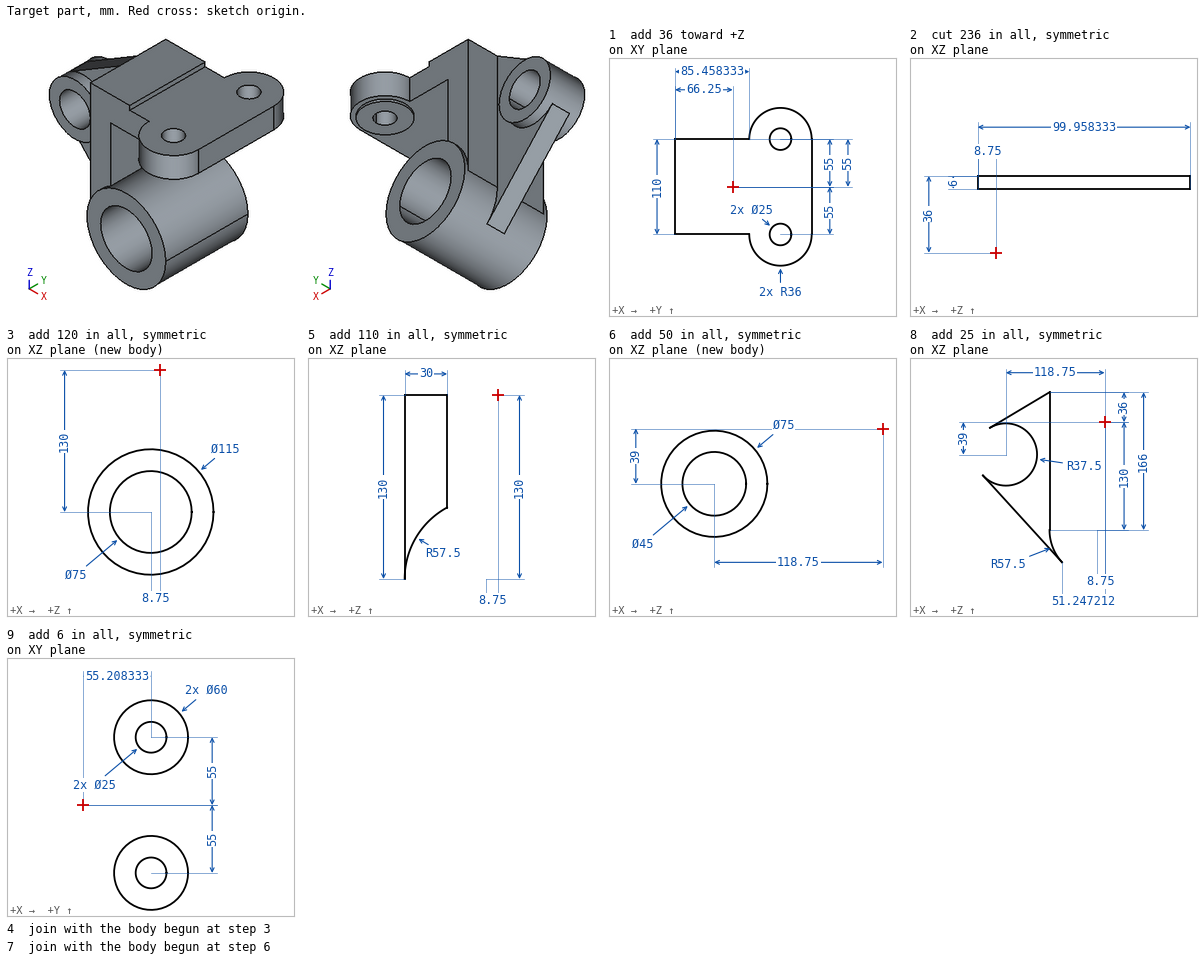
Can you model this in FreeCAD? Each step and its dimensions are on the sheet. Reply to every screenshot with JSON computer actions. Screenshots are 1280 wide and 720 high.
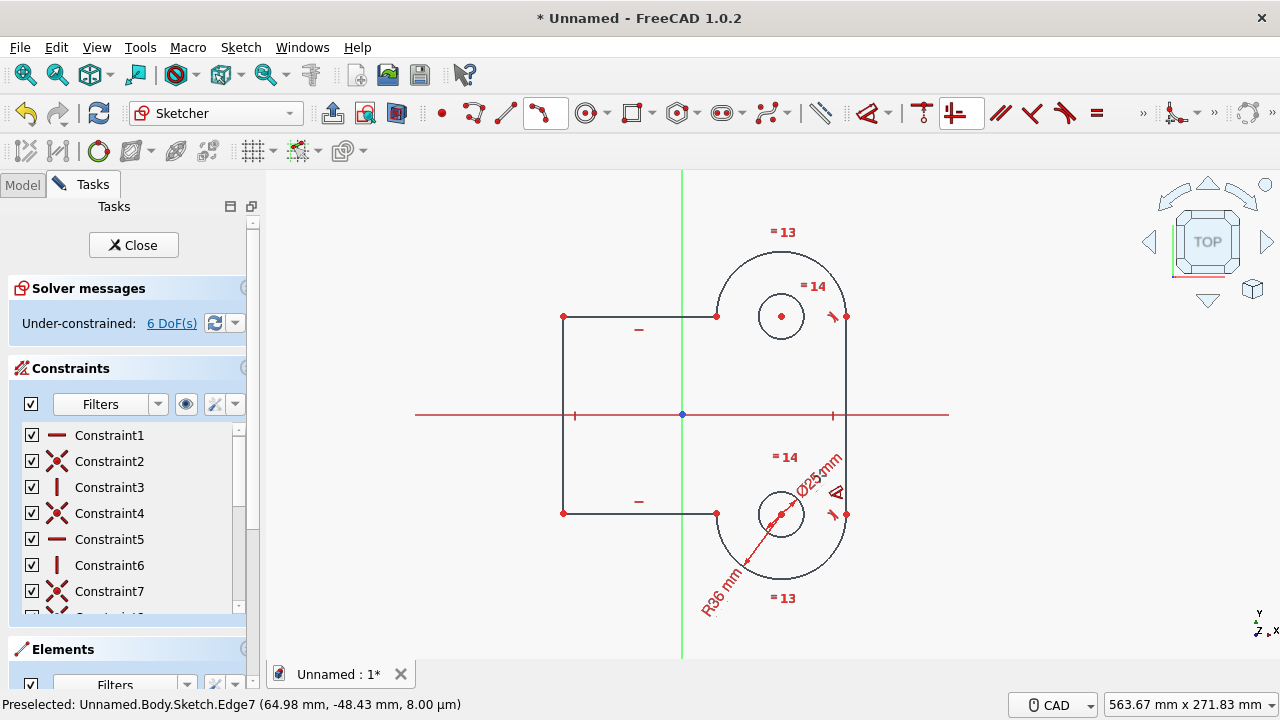
{"action": "left_click", "coordinate": [781, 514]}
{"action": "left_click", "coordinate": [815, 441]}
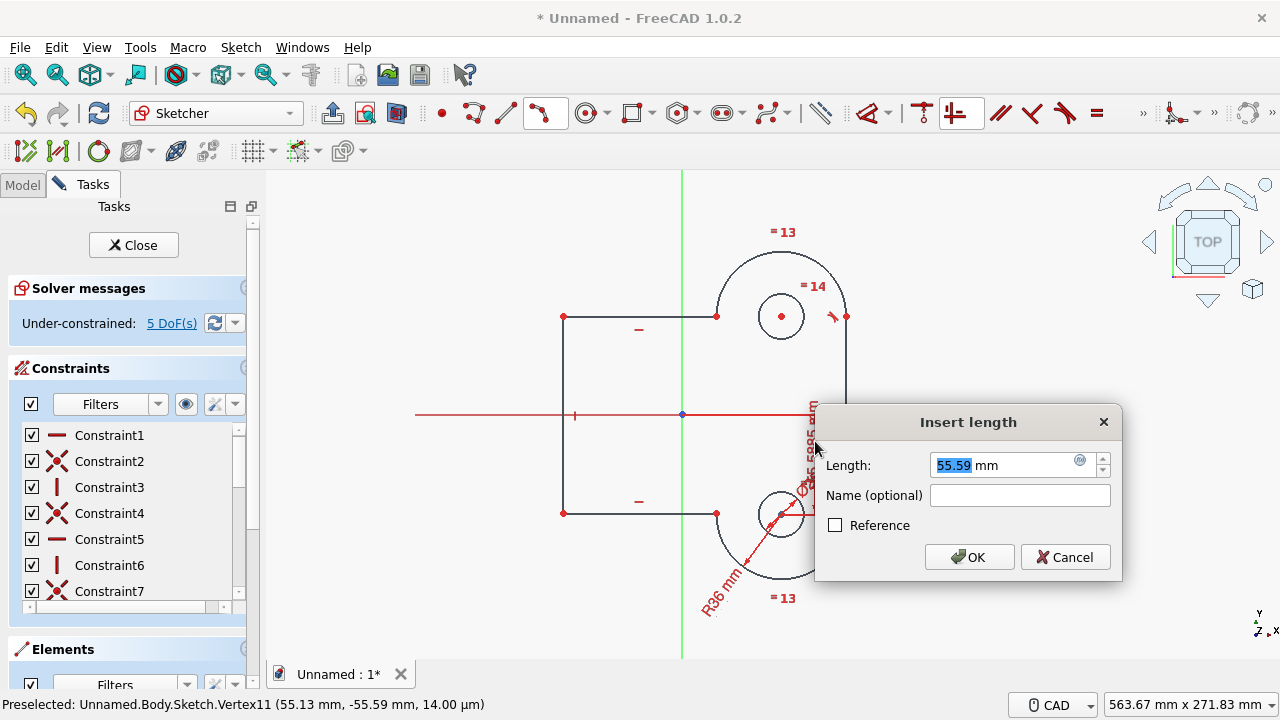
{"action": "type", "text": "55"}
{"action": "key", "text": "Return"}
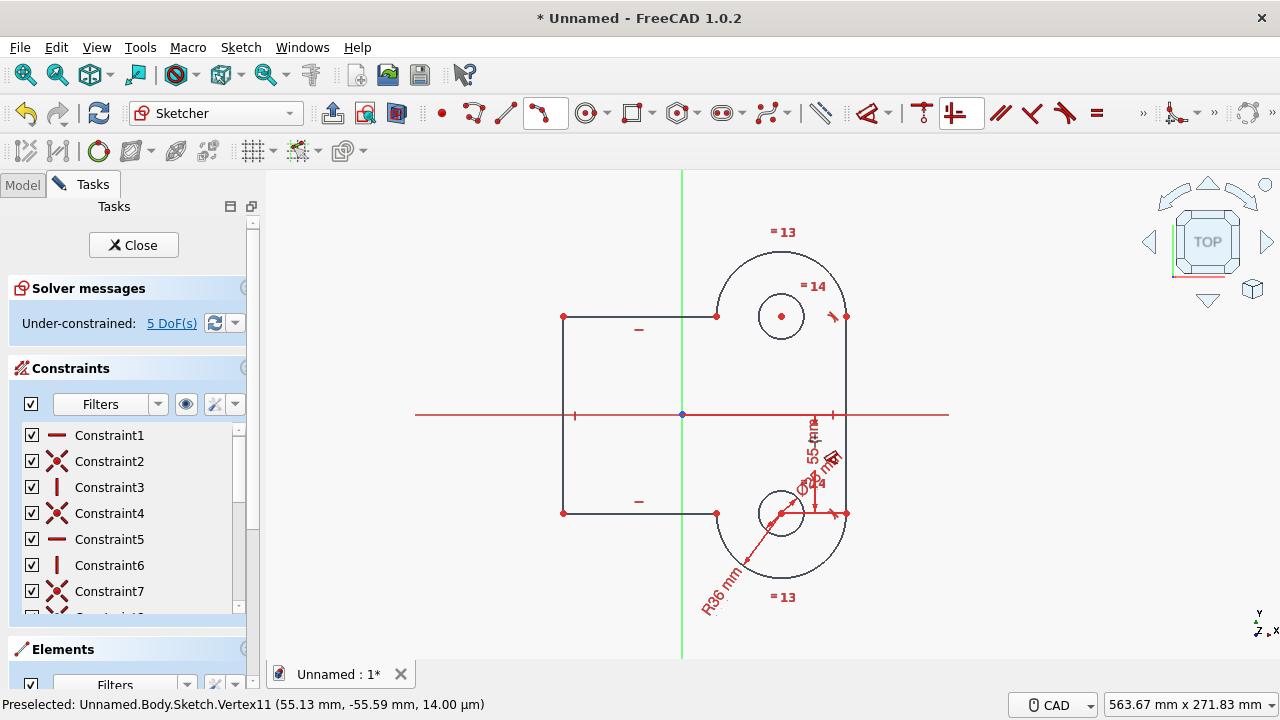
{"action": "left_click", "coordinate": [781, 317]}
{"action": "left_click", "coordinate": [815, 366]}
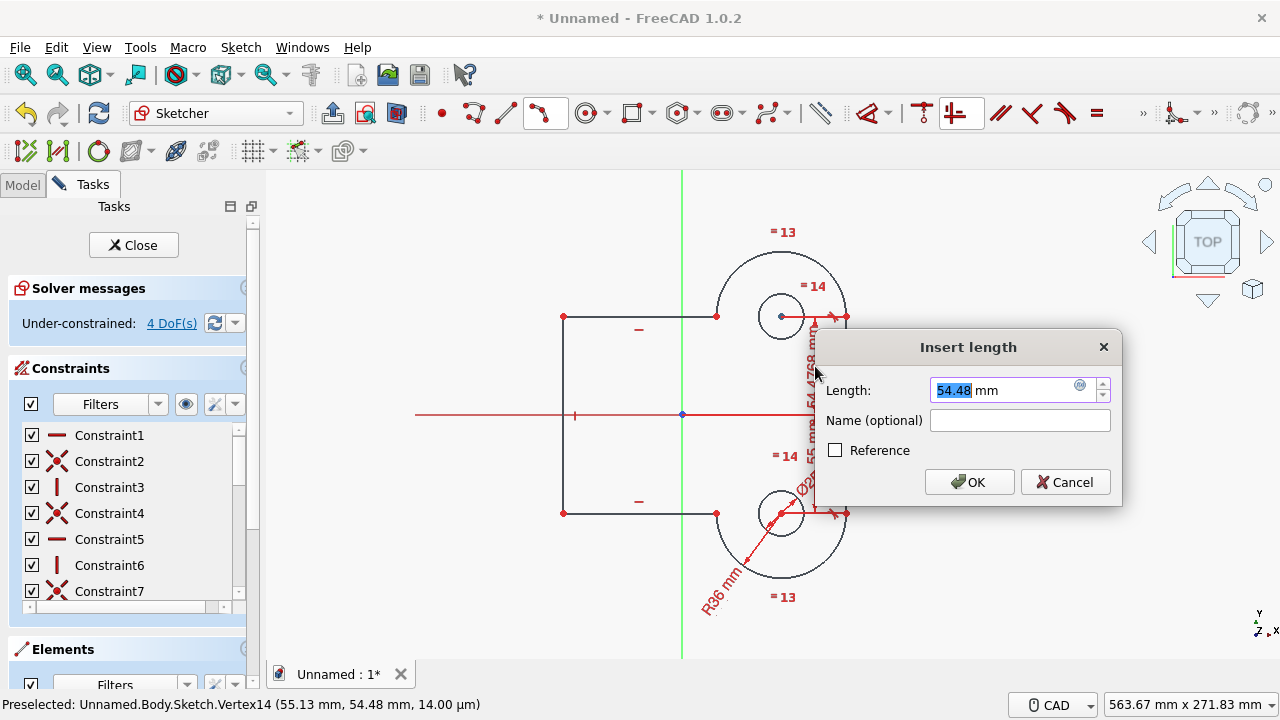
{"action": "type", "text": "55"}
{"action": "key", "text": "Return"}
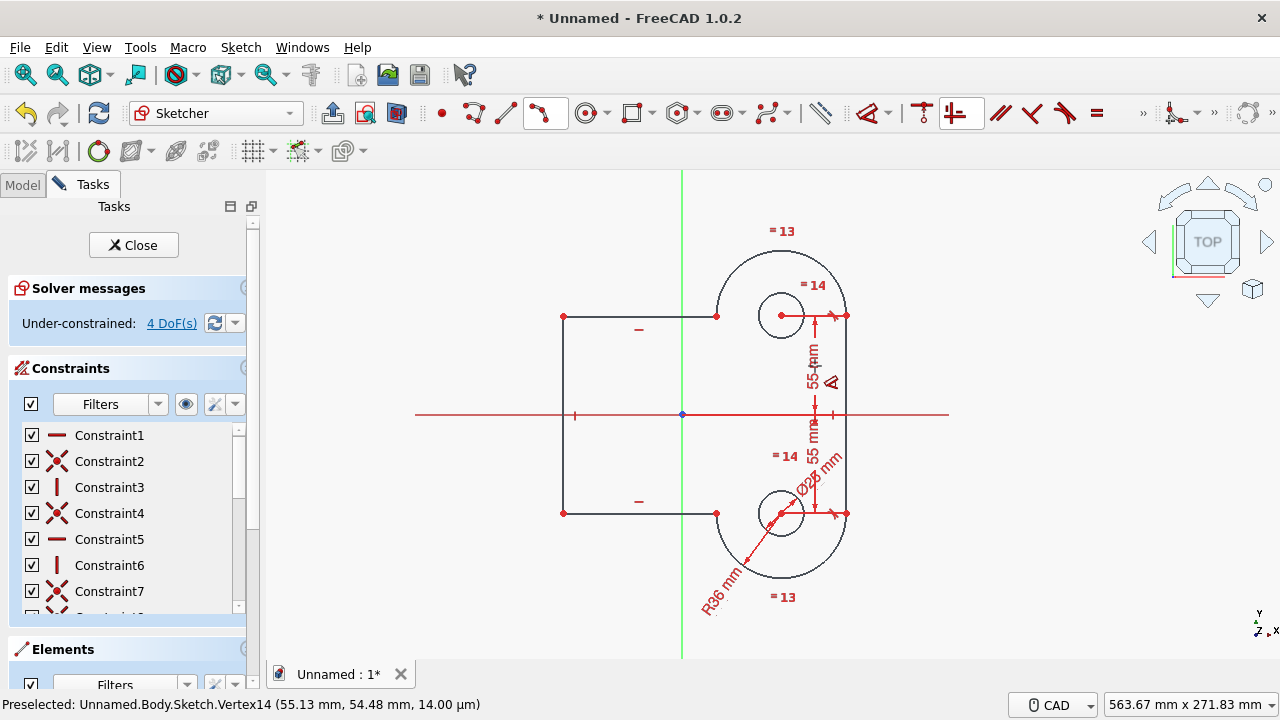
{"action": "left_click", "coordinate": [563, 376]}
{"action": "left_click", "coordinate": [529, 370]}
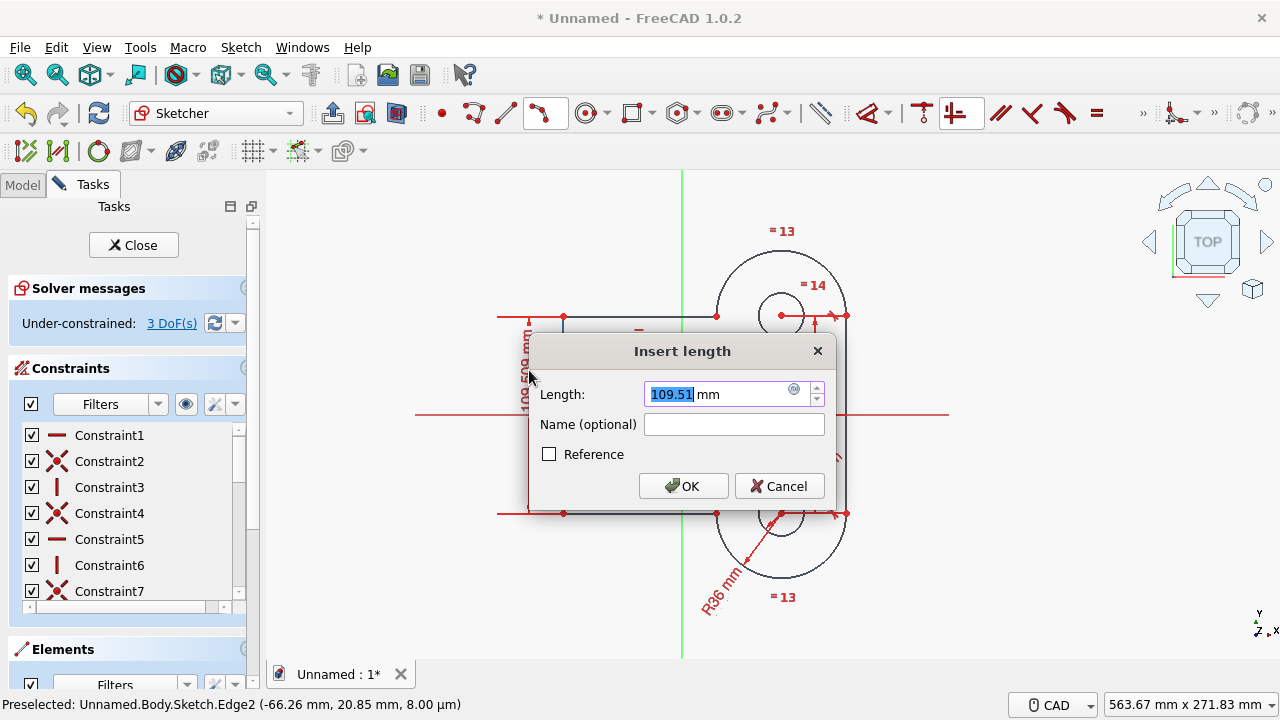
{"action": "type", "text": "110"}
{"action": "key", "text": "Return"}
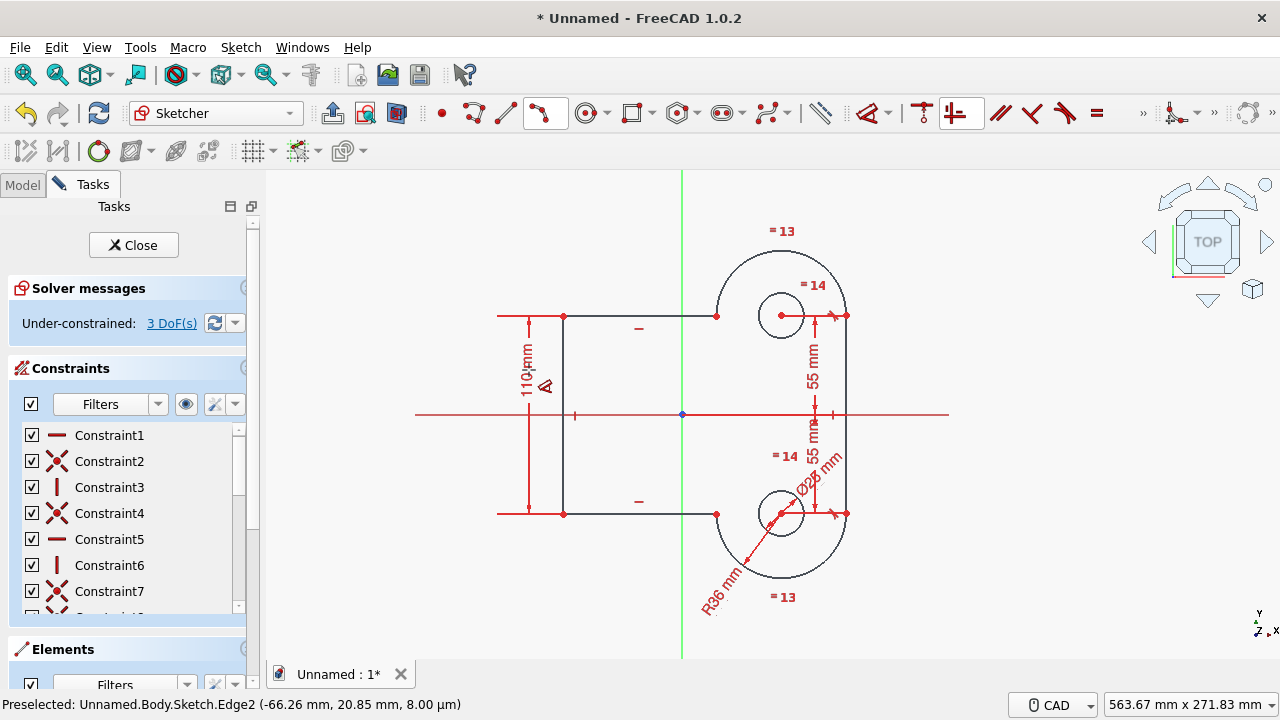
{"action": "left_click", "coordinate": [717, 316]}
{"action": "left_click", "coordinate": [648, 365]}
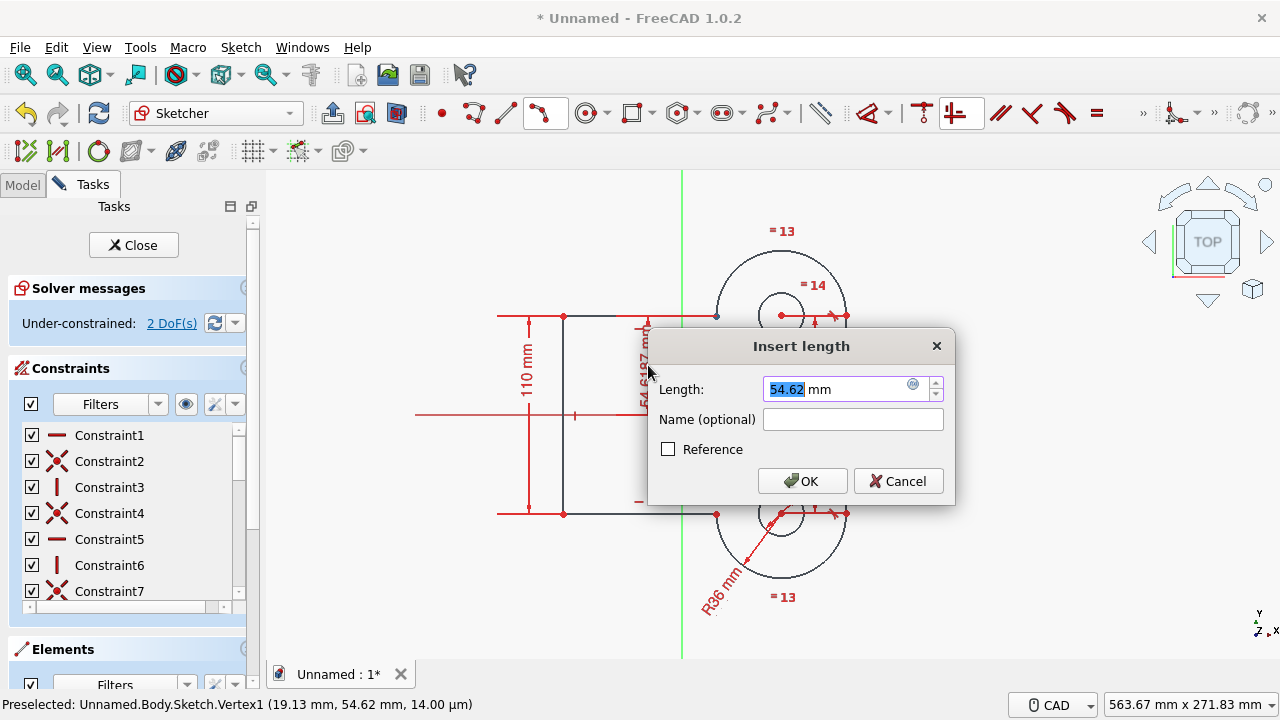
{"action": "type", "text": "55"}
{"action": "key", "text": "Return"}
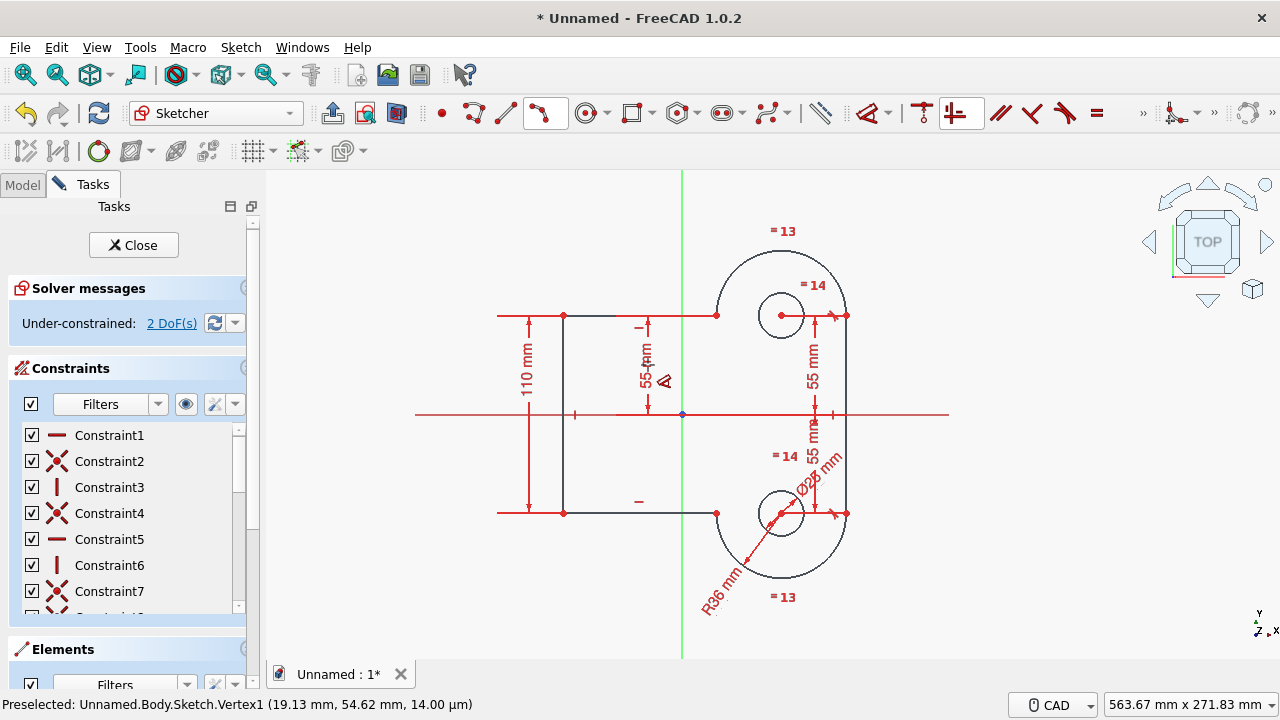
{"action": "left_click", "coordinate": [563, 316]}
{"action": "left_click", "coordinate": [623, 282]}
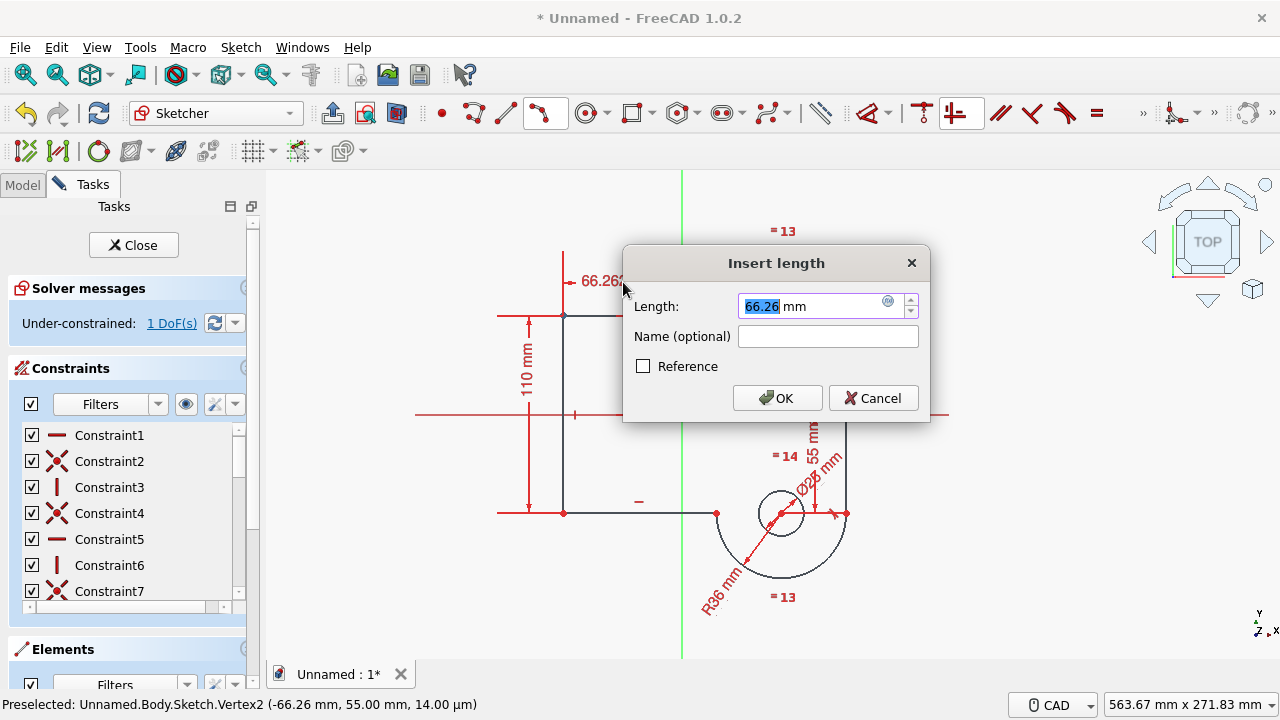
{"action": "type", "text": "66.25"}
{"action": "key", "text": "Return"}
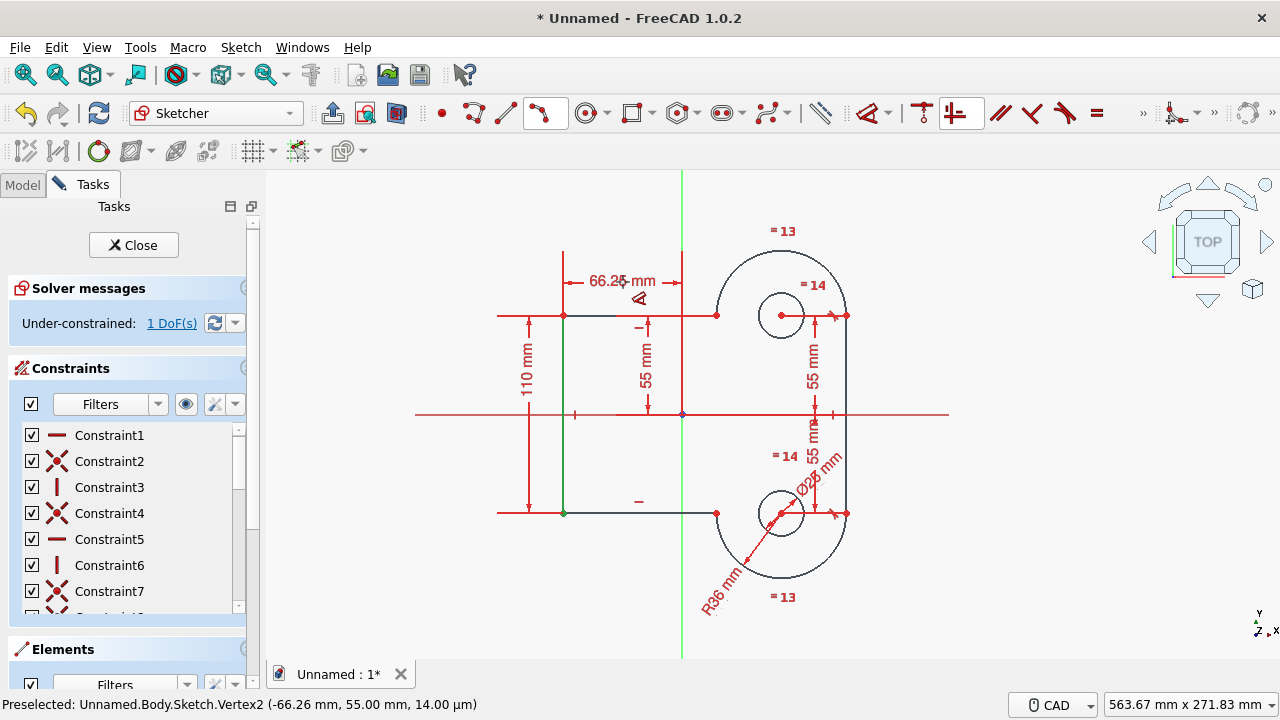
{"action": "left_click", "coordinate": [671, 316]}
{"action": "left_click", "coordinate": [640, 258]}